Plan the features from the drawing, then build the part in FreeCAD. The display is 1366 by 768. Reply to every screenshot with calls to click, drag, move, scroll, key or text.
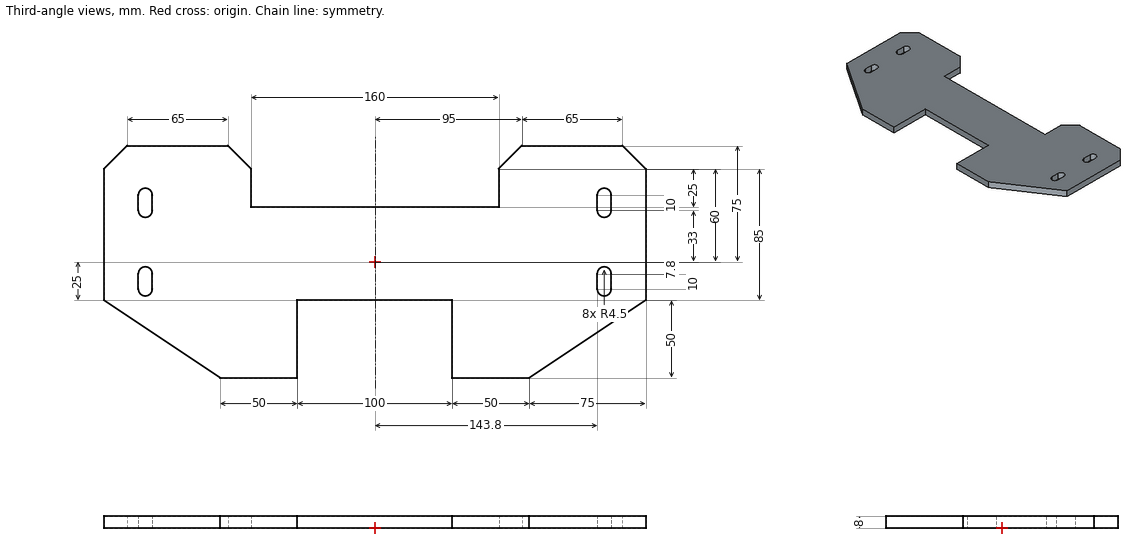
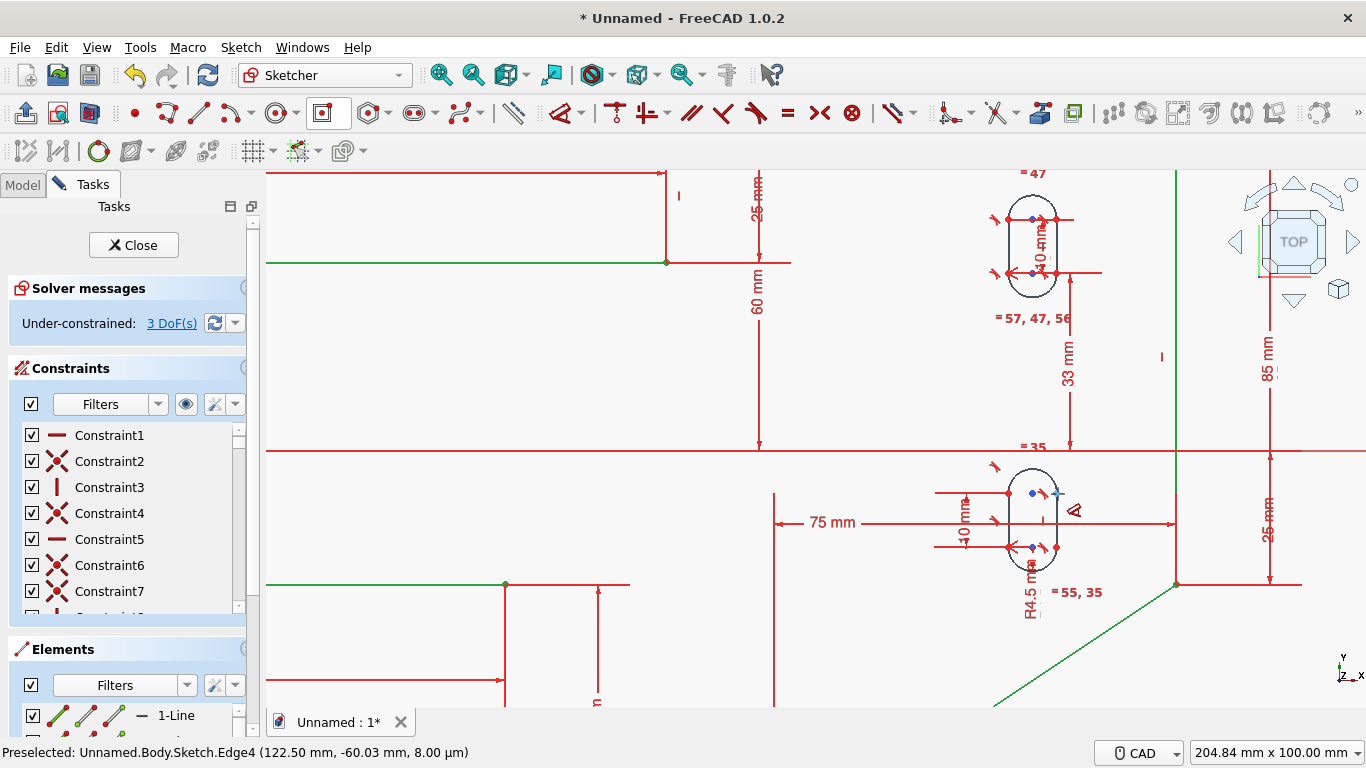
click(1057, 493)
click(1091, 472)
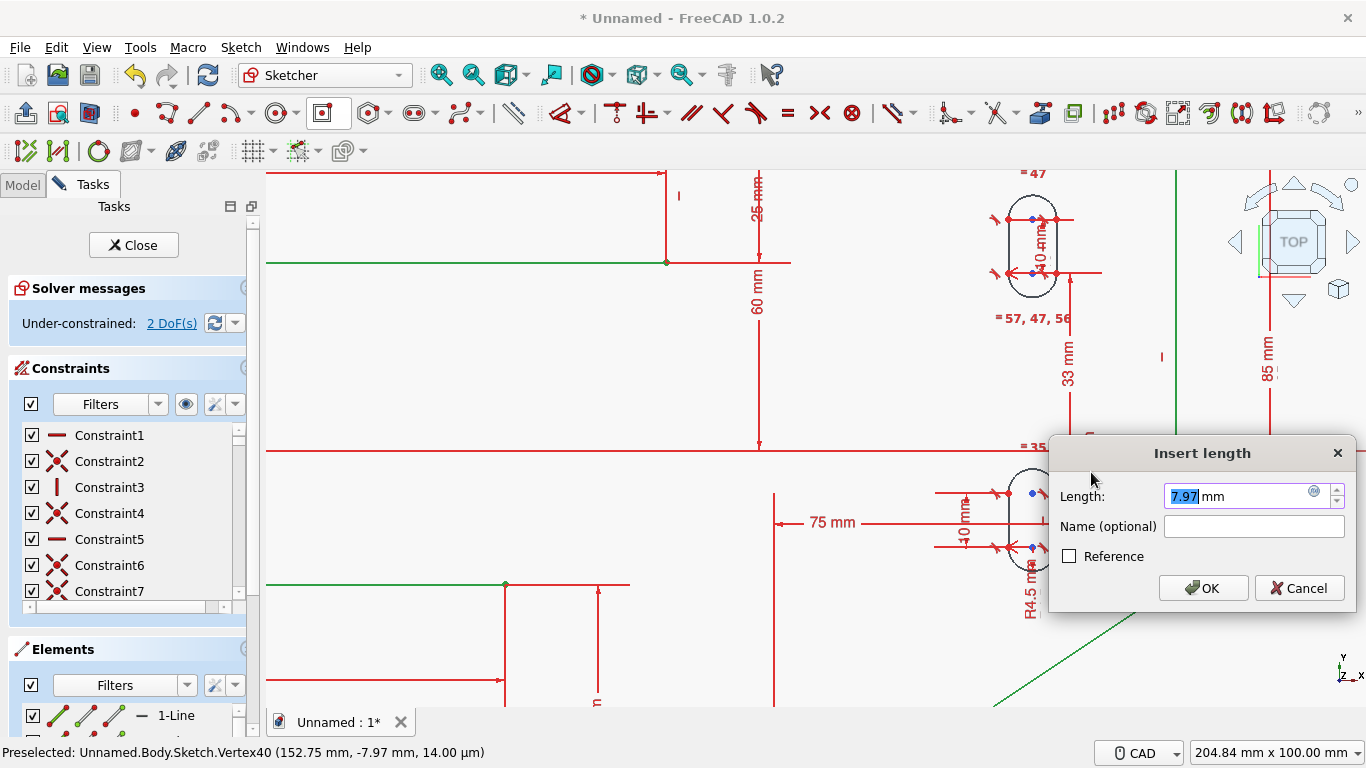
text(7.8)
key(Return)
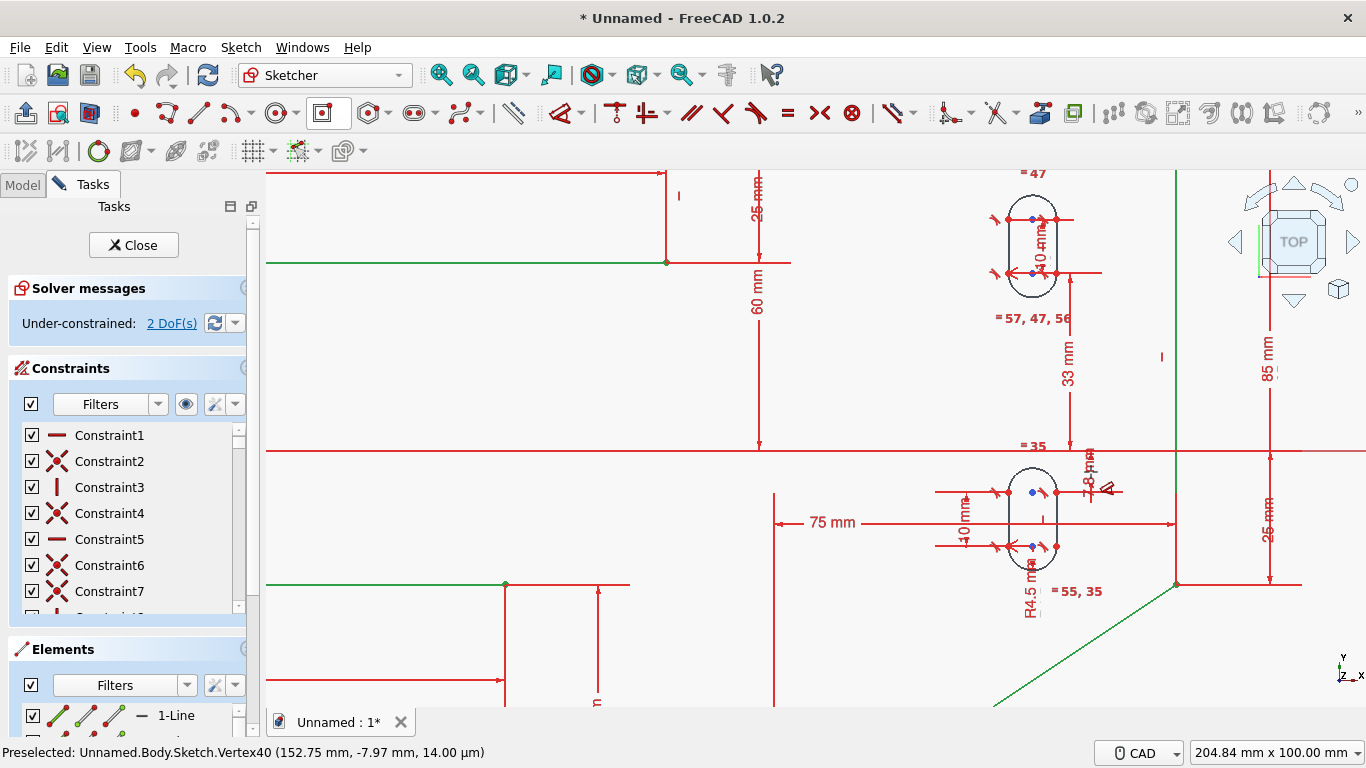
click(1009, 546)
click(651, 580)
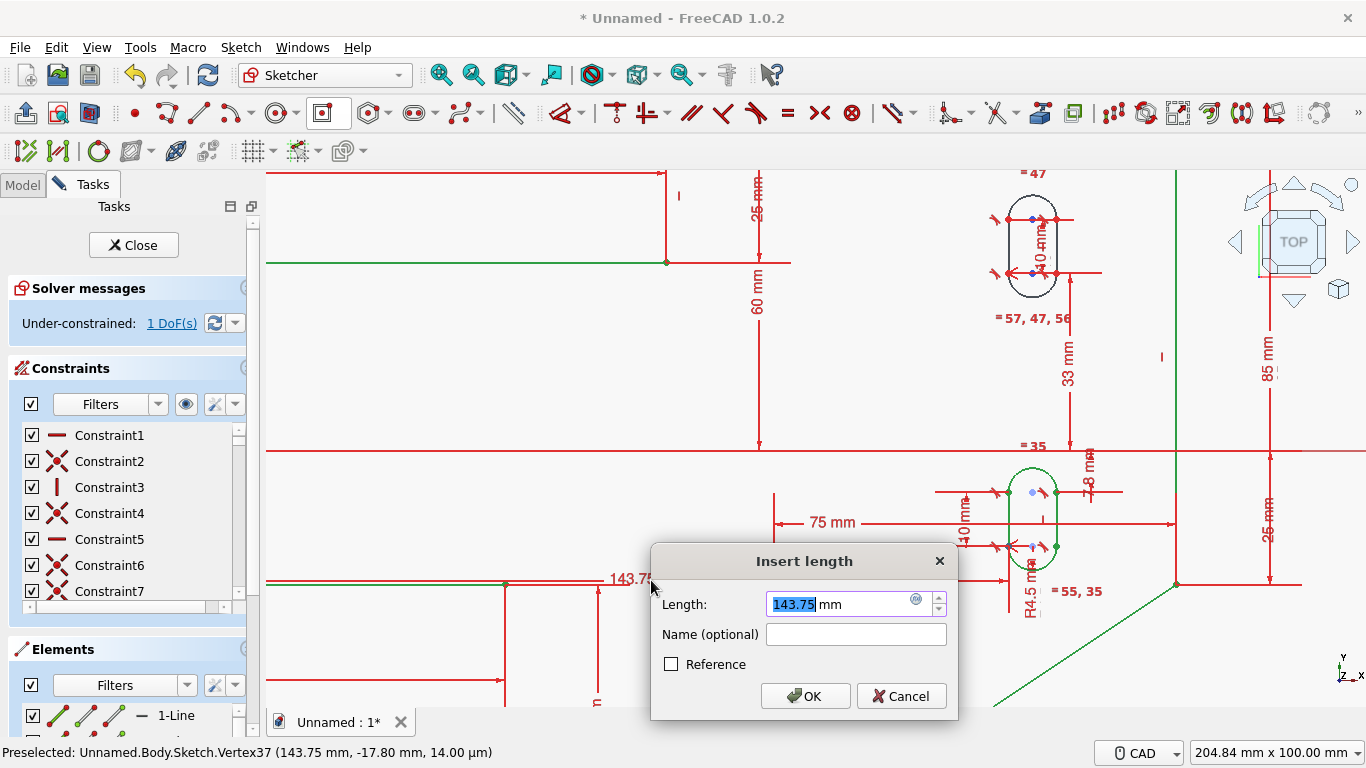
text(143.8)
key(Return)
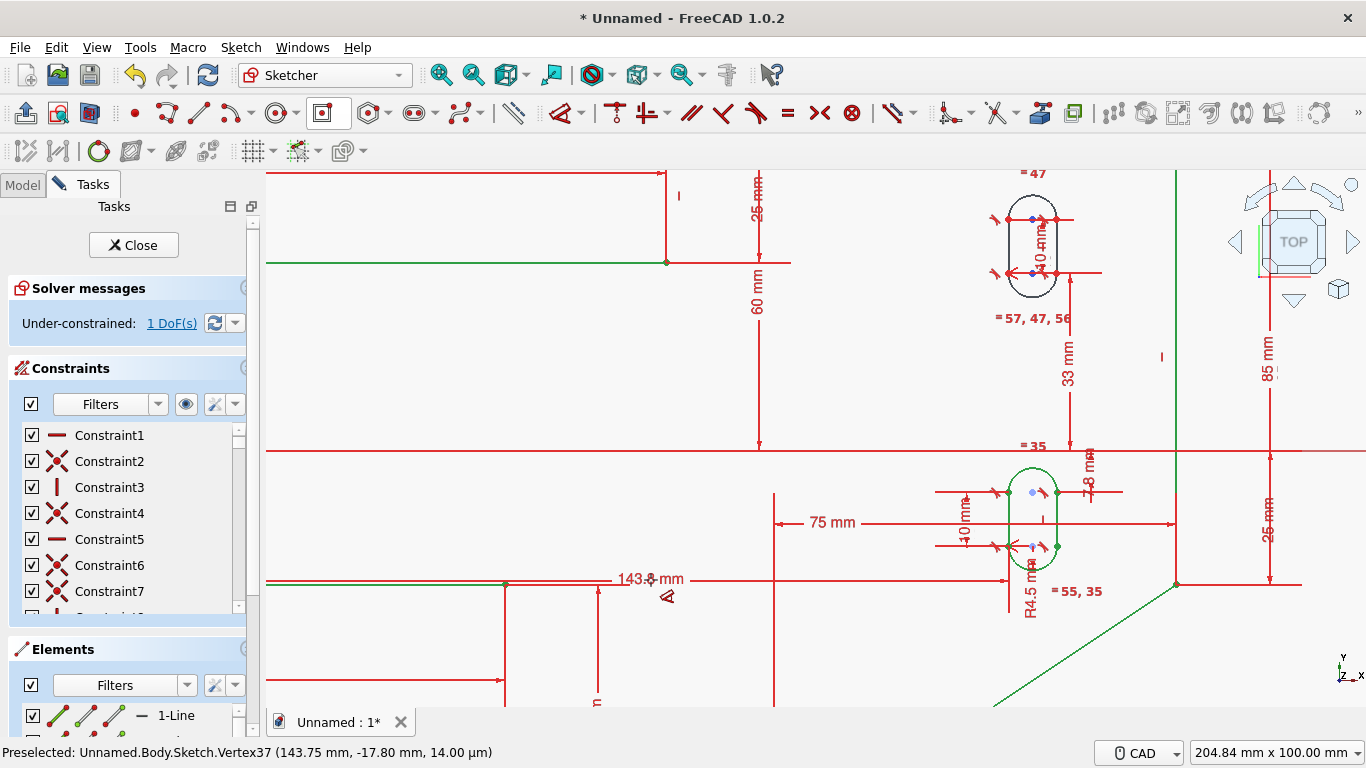
click(1009, 273)
click(651, 239)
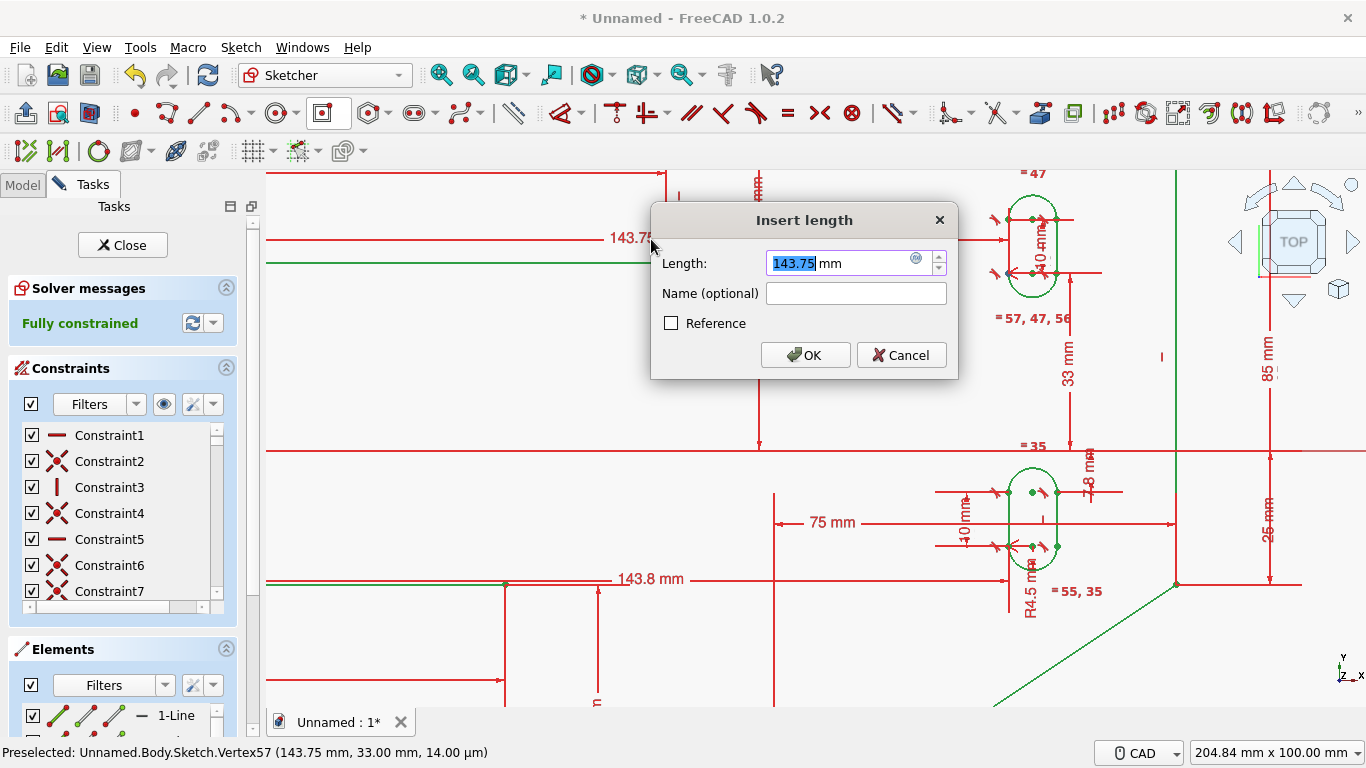
text(143.8)
key(Return)
key(Escape)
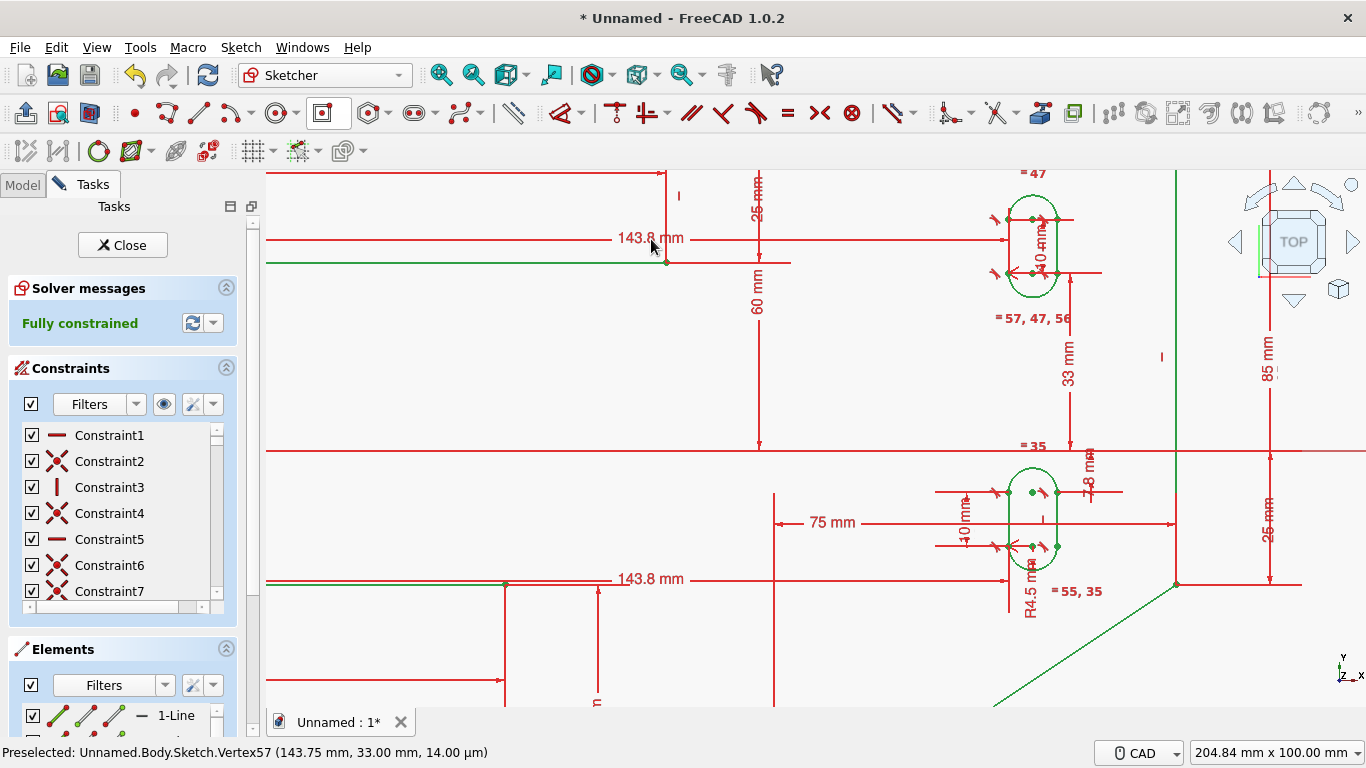
click(123, 245)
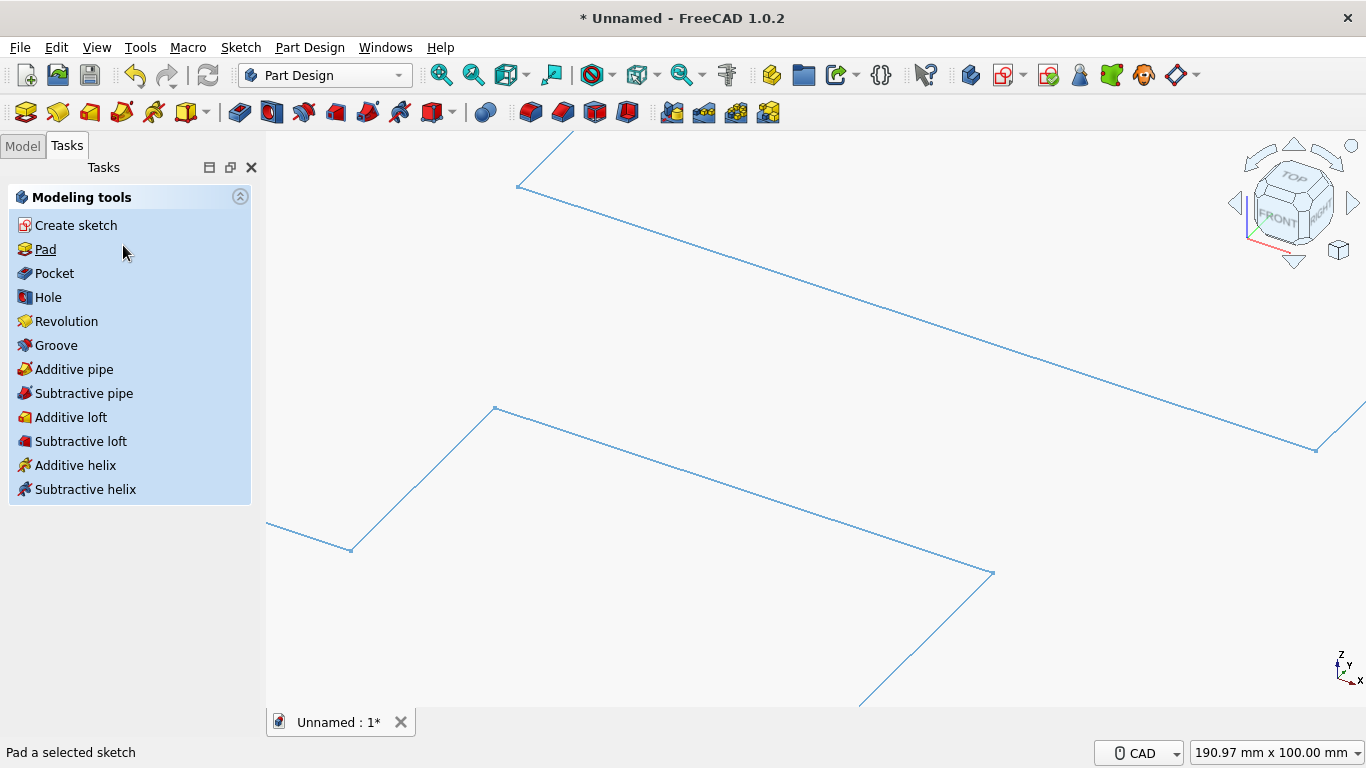
click(26, 112)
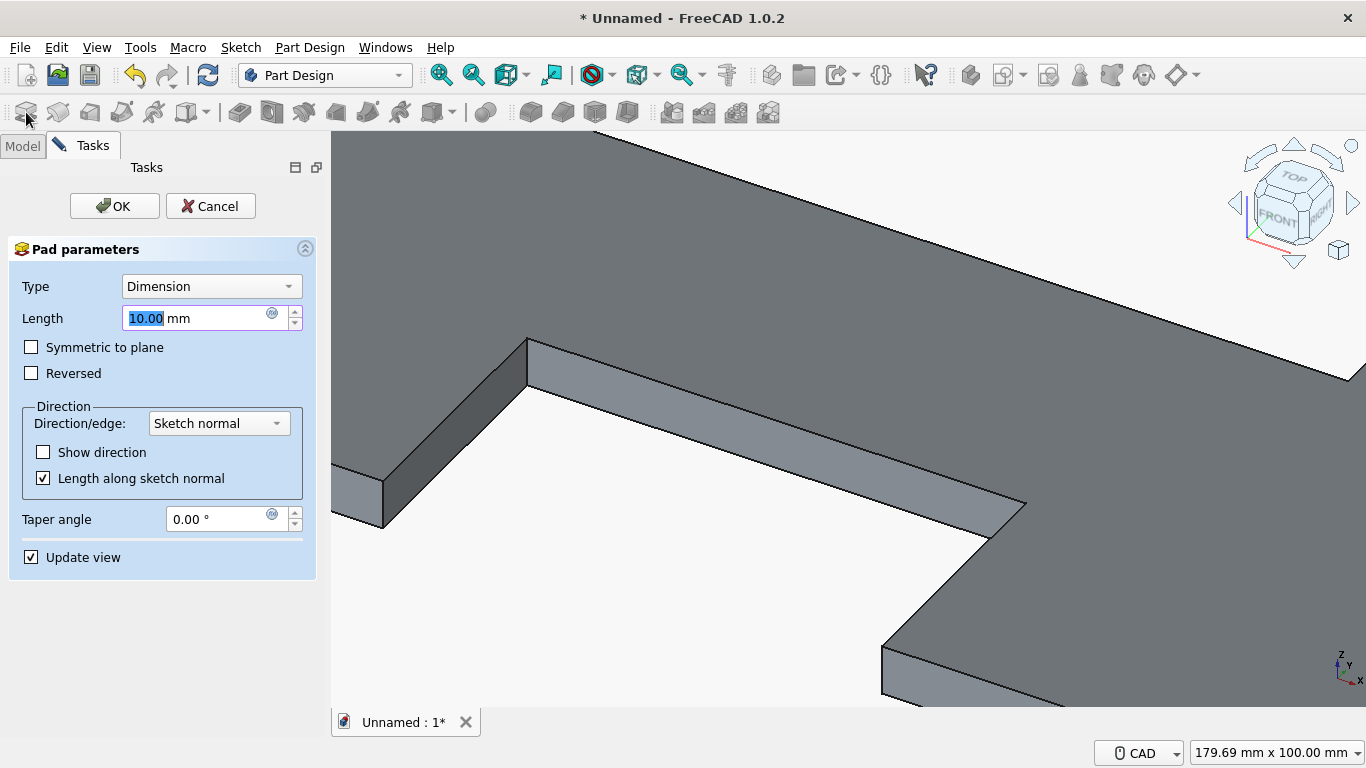
text(8)
key(Tab)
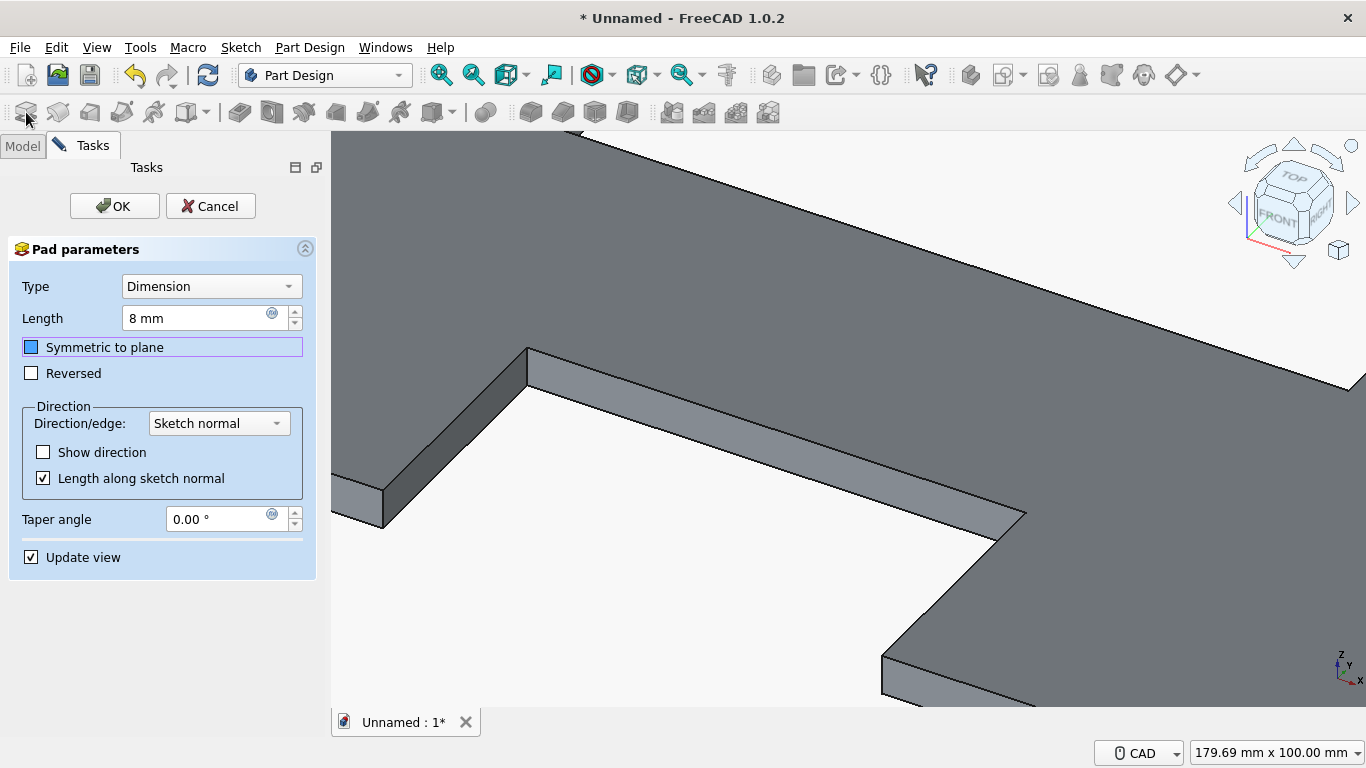
click(115, 206)